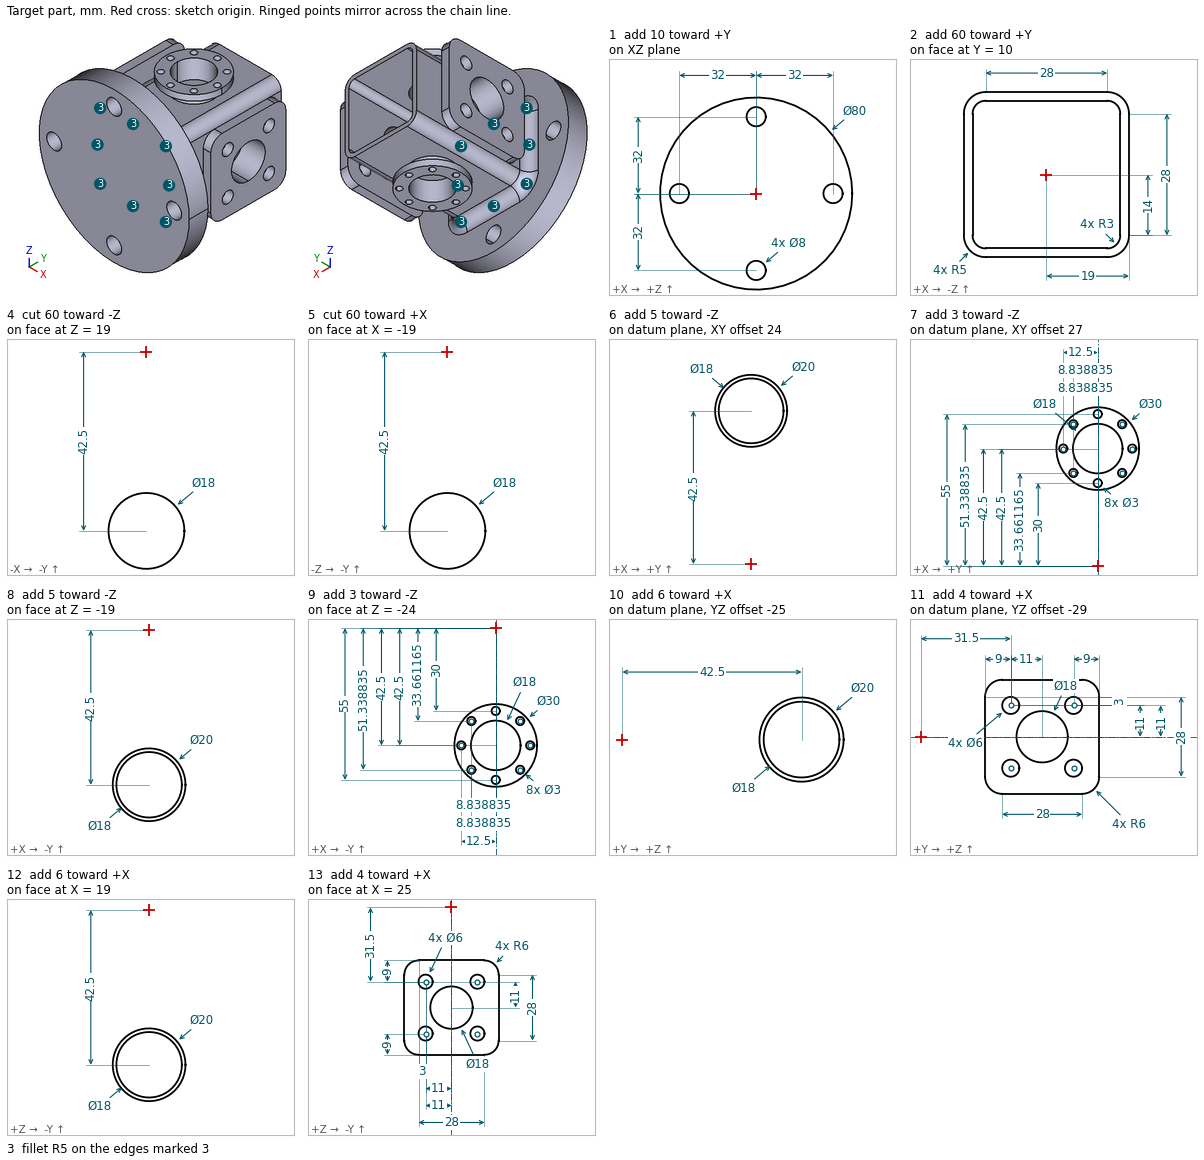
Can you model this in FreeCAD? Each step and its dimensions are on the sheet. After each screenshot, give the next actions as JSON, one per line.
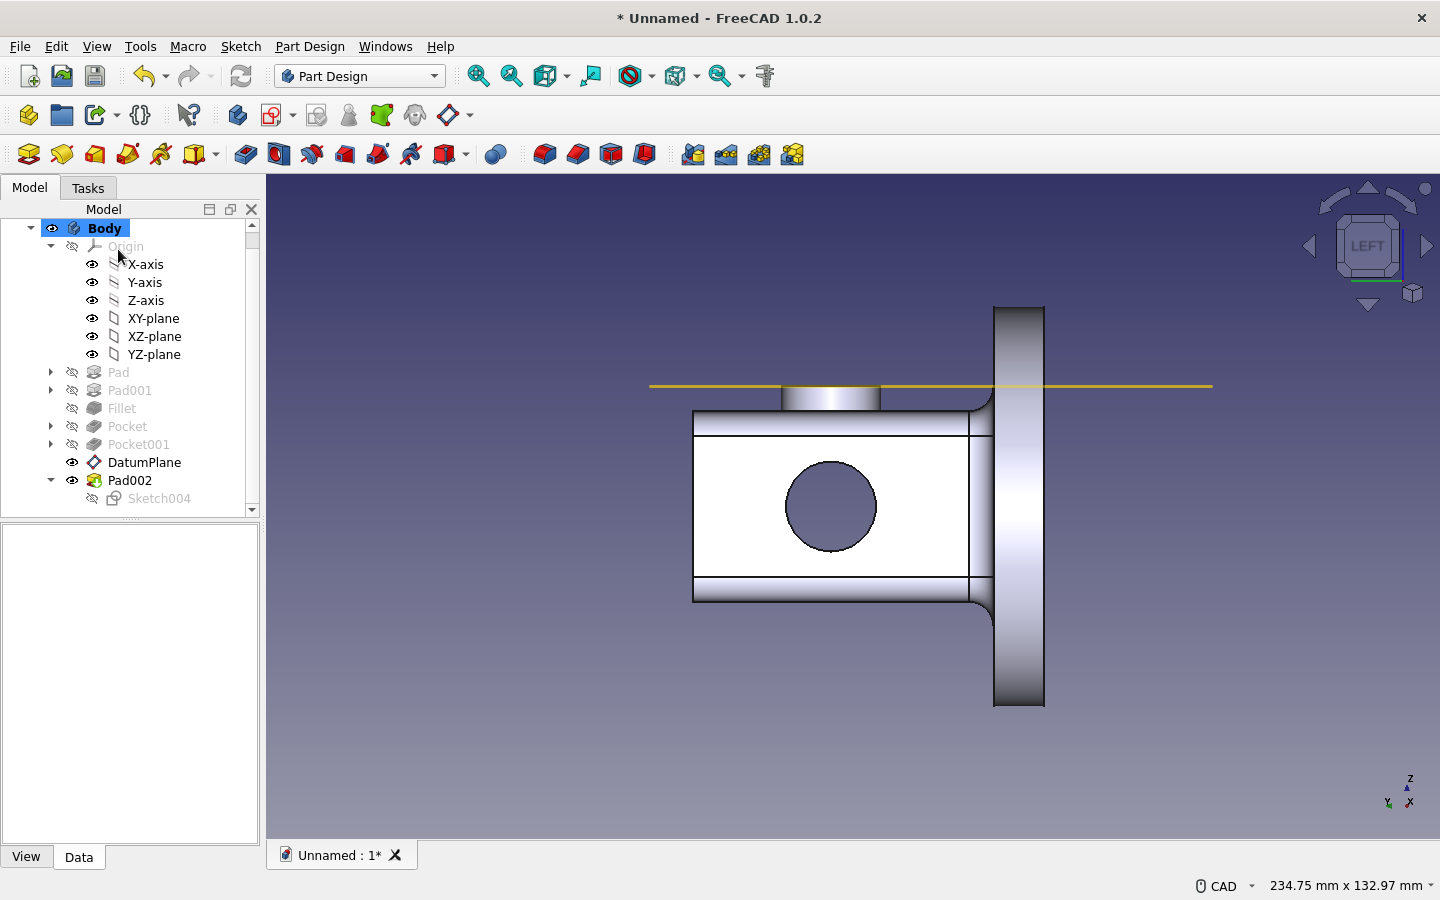
{"action": "left_click", "coordinate": [117, 462]}
{"action": "key", "text": "space"}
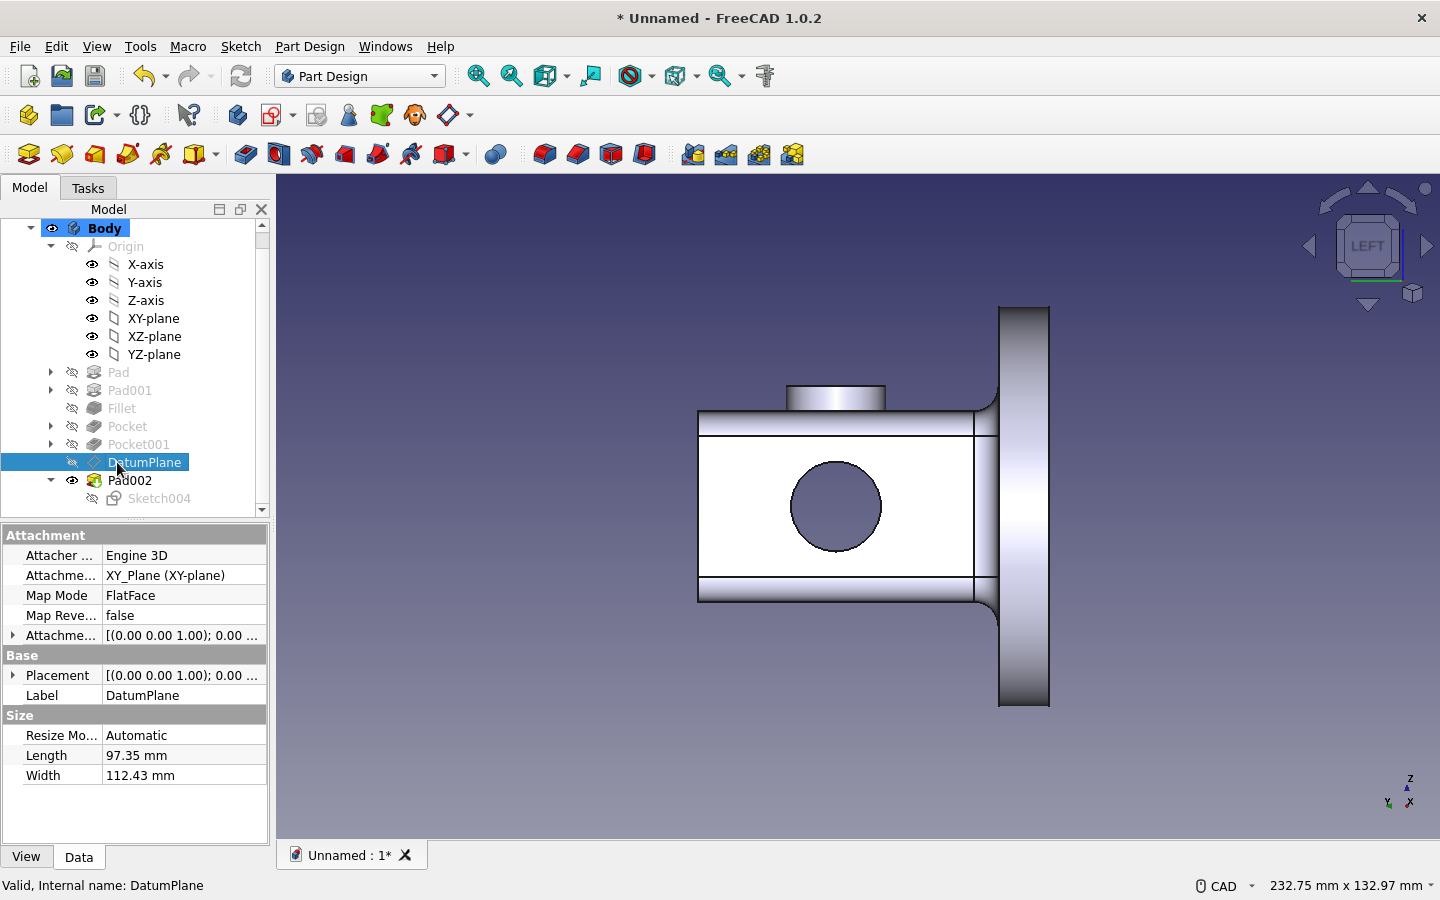
{"action": "left_click", "coordinate": [137, 318]}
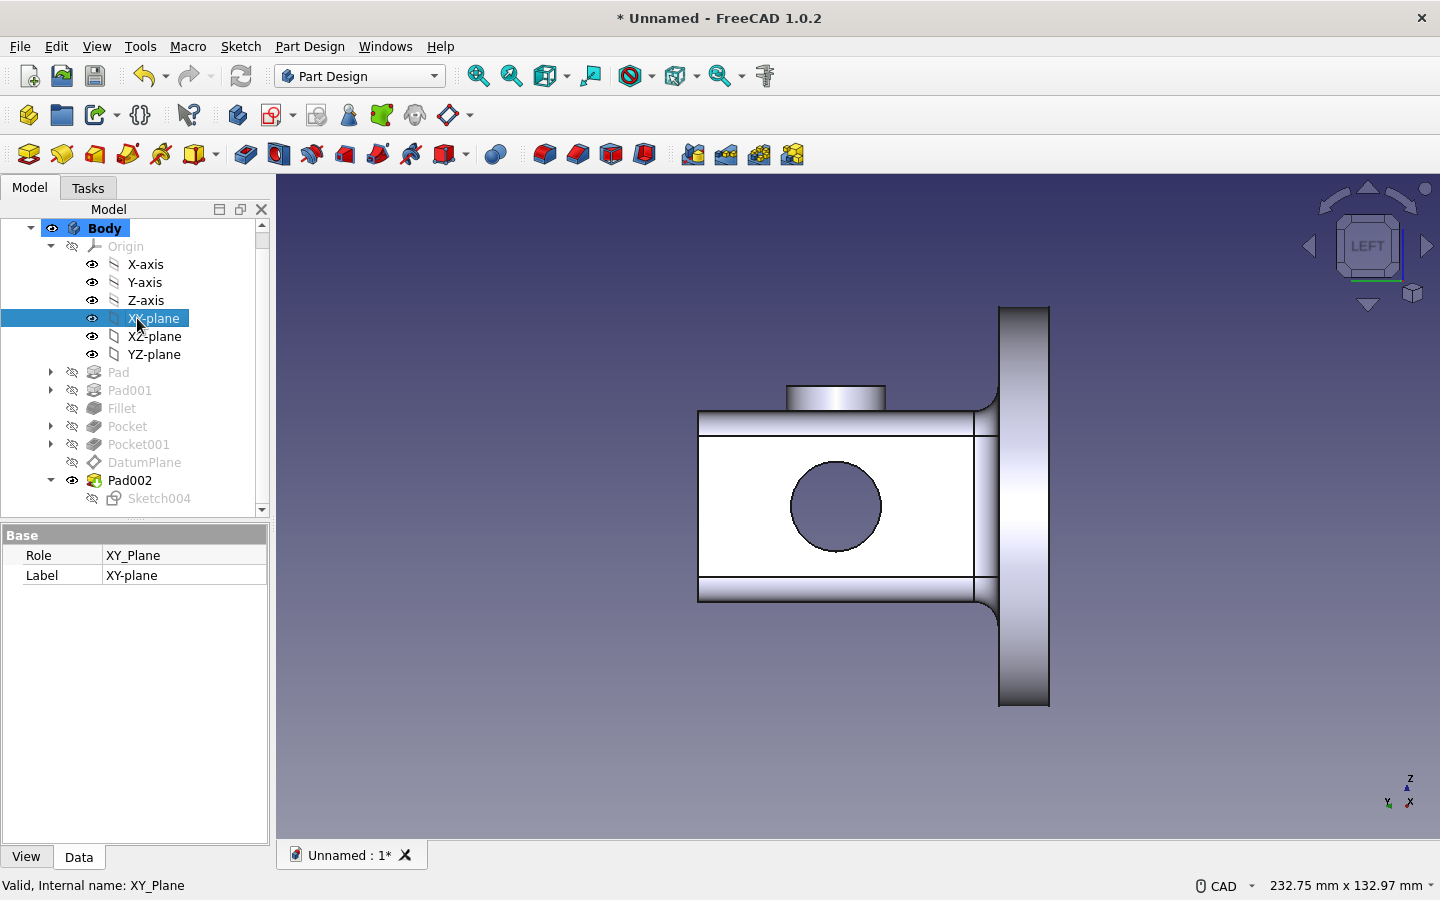
{"action": "left_click", "coordinate": [448, 116]}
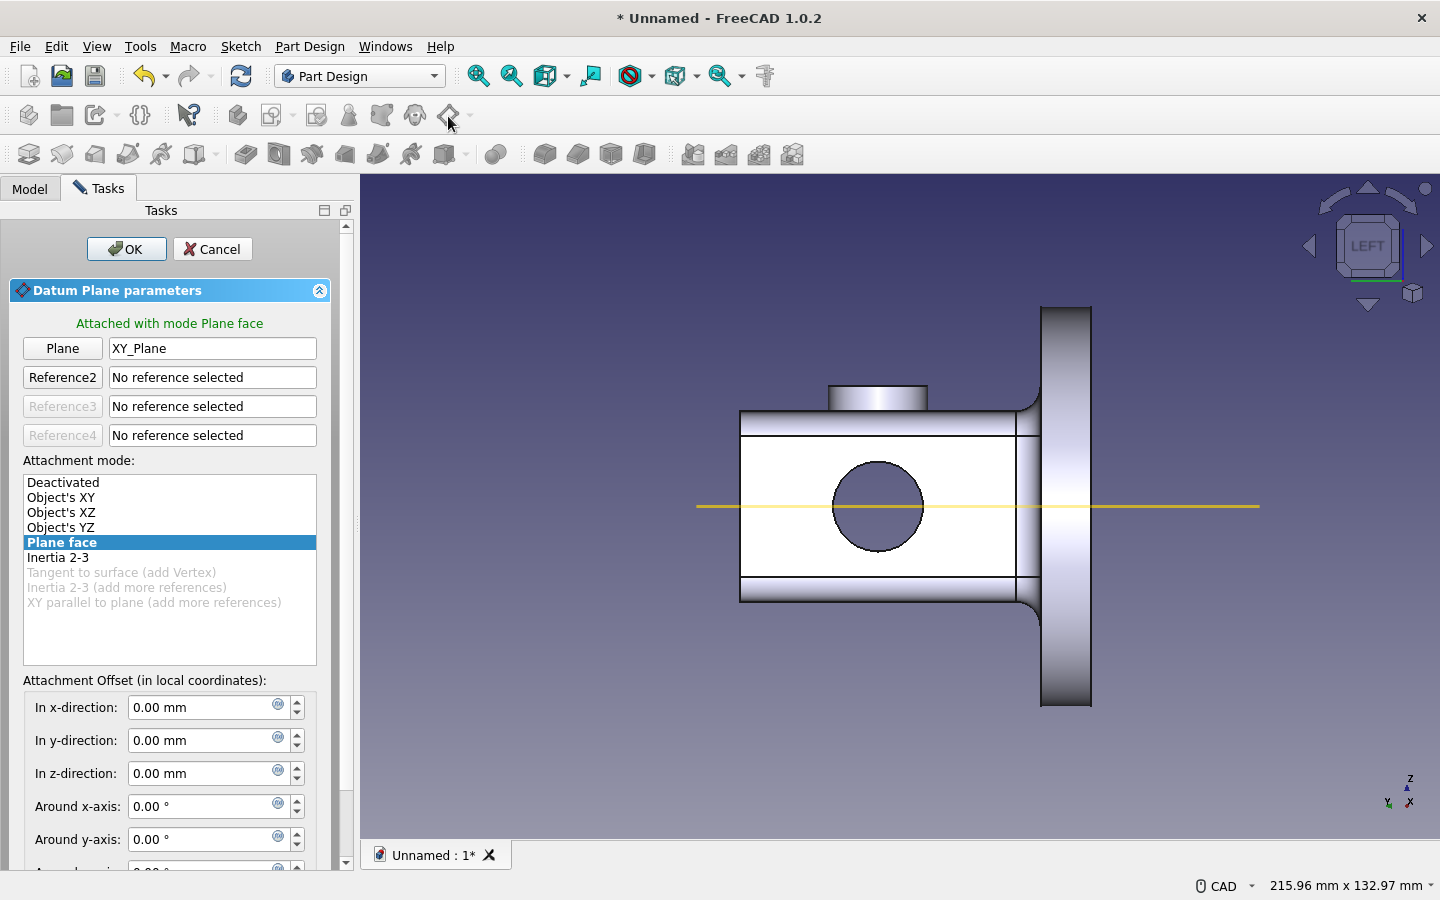
{"action": "triple_click", "coordinate": [210, 774]}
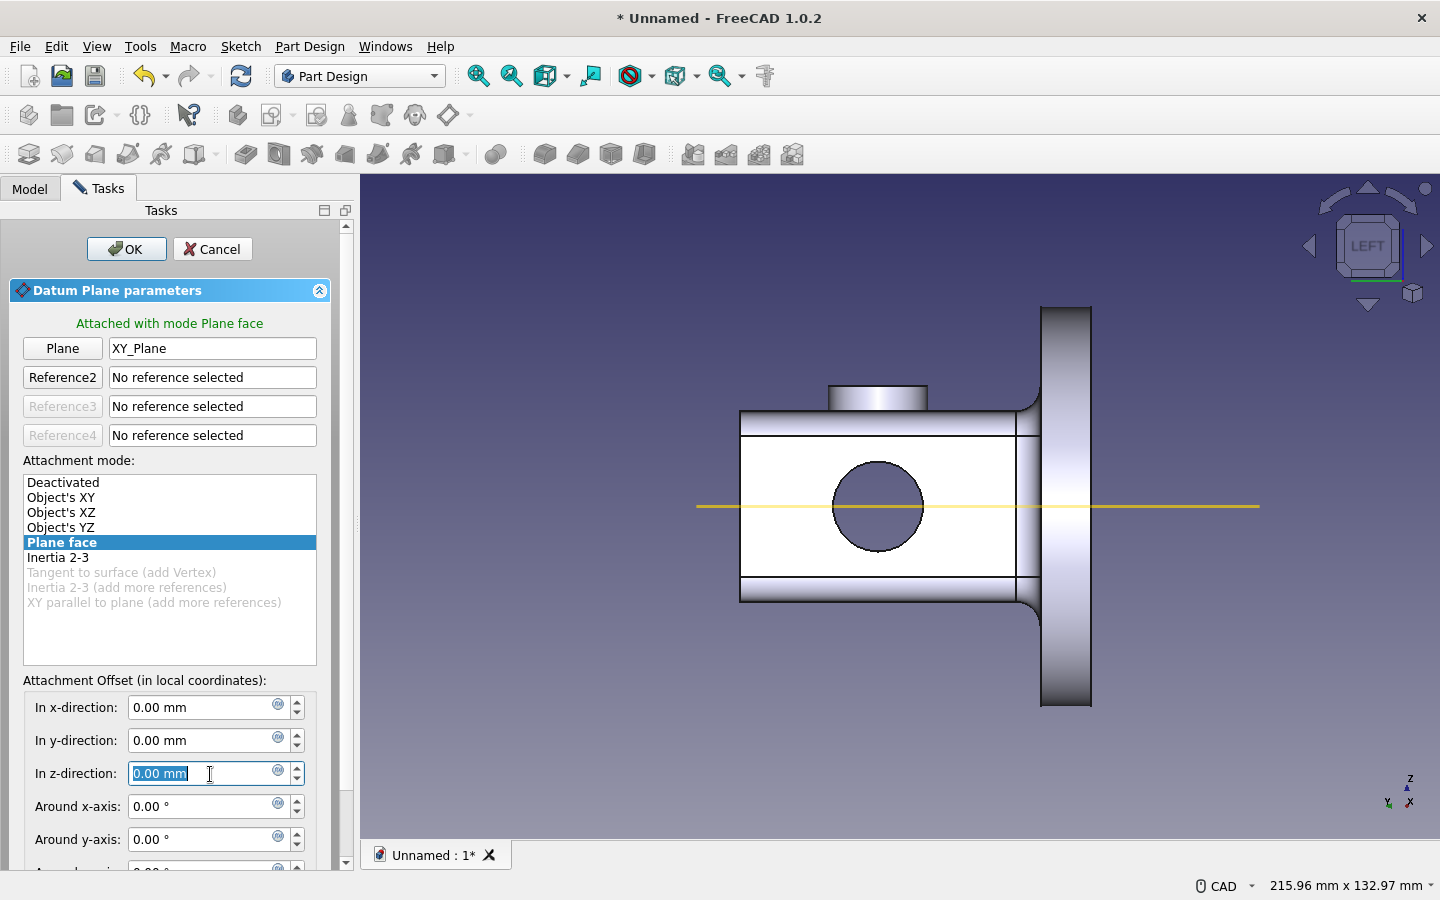
{"action": "type", "text": "27"}
{"action": "key", "text": "Tab"}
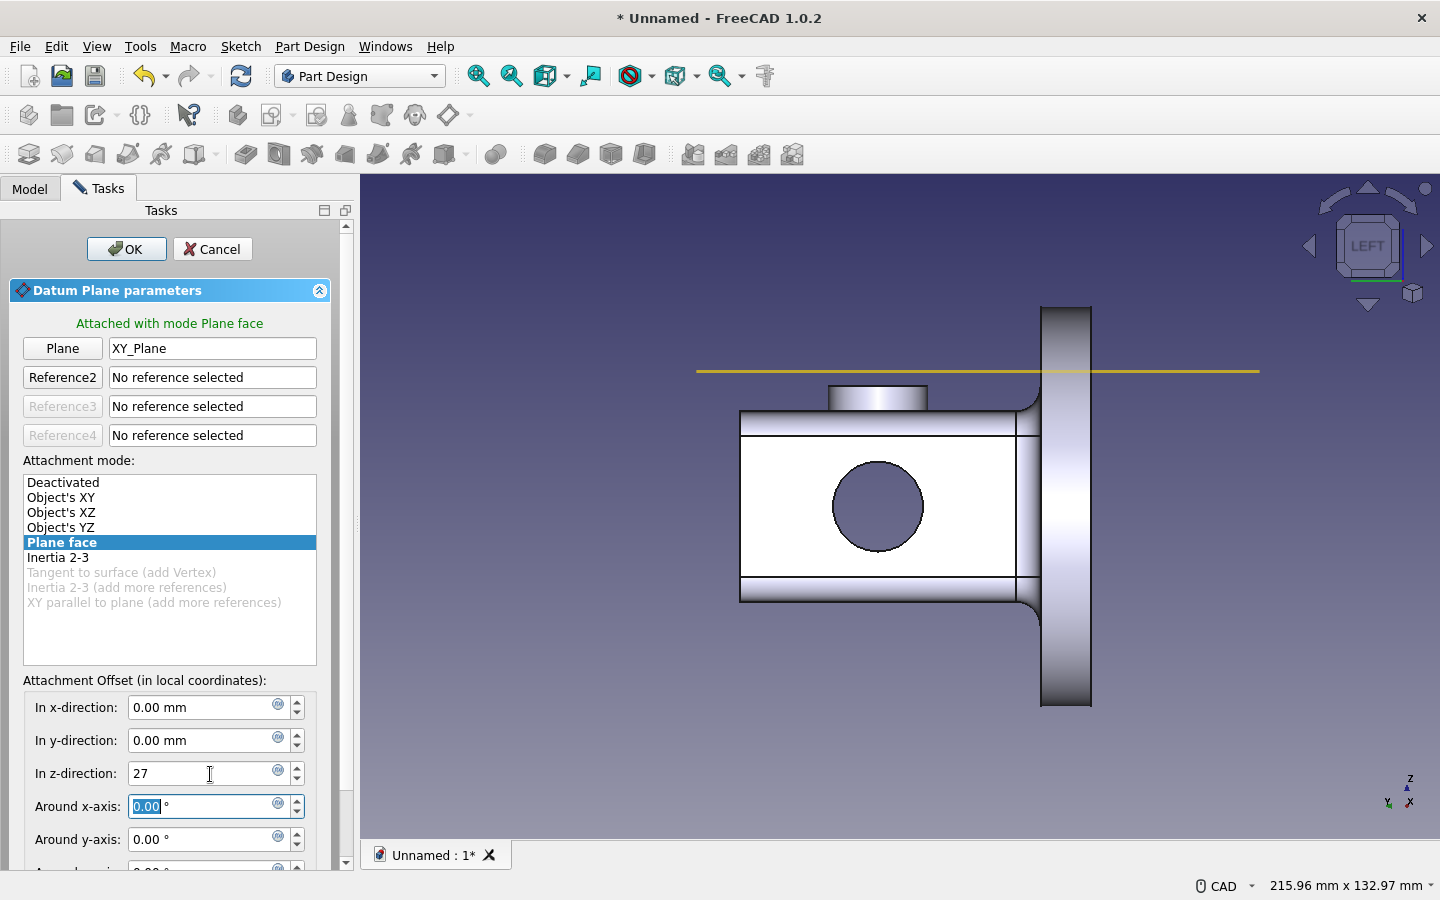
{"action": "left_click", "coordinate": [127, 249]}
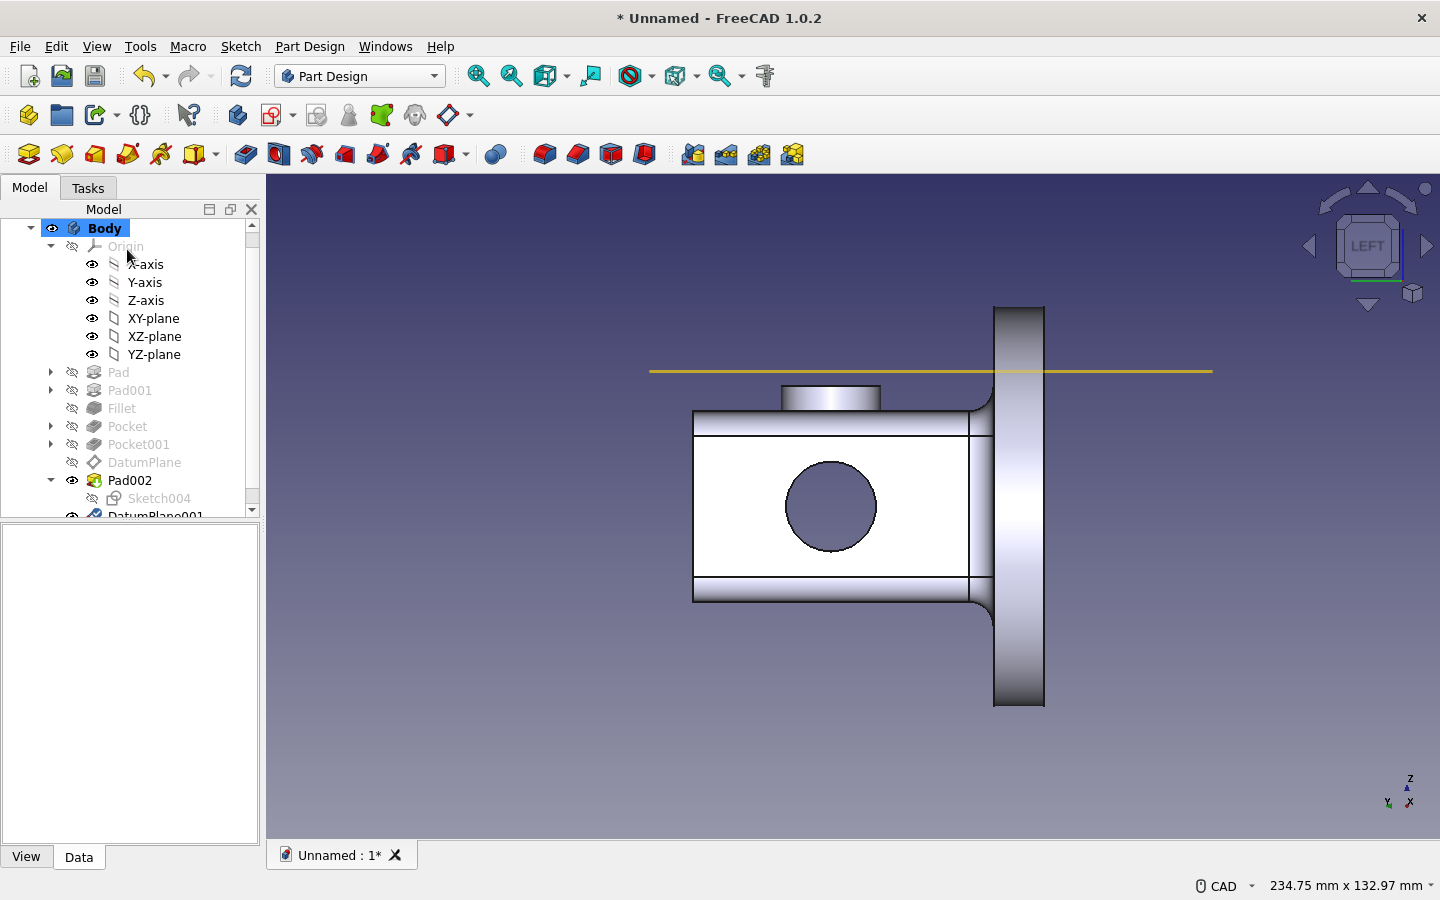
{"action": "left_click", "coordinate": [117, 516]}